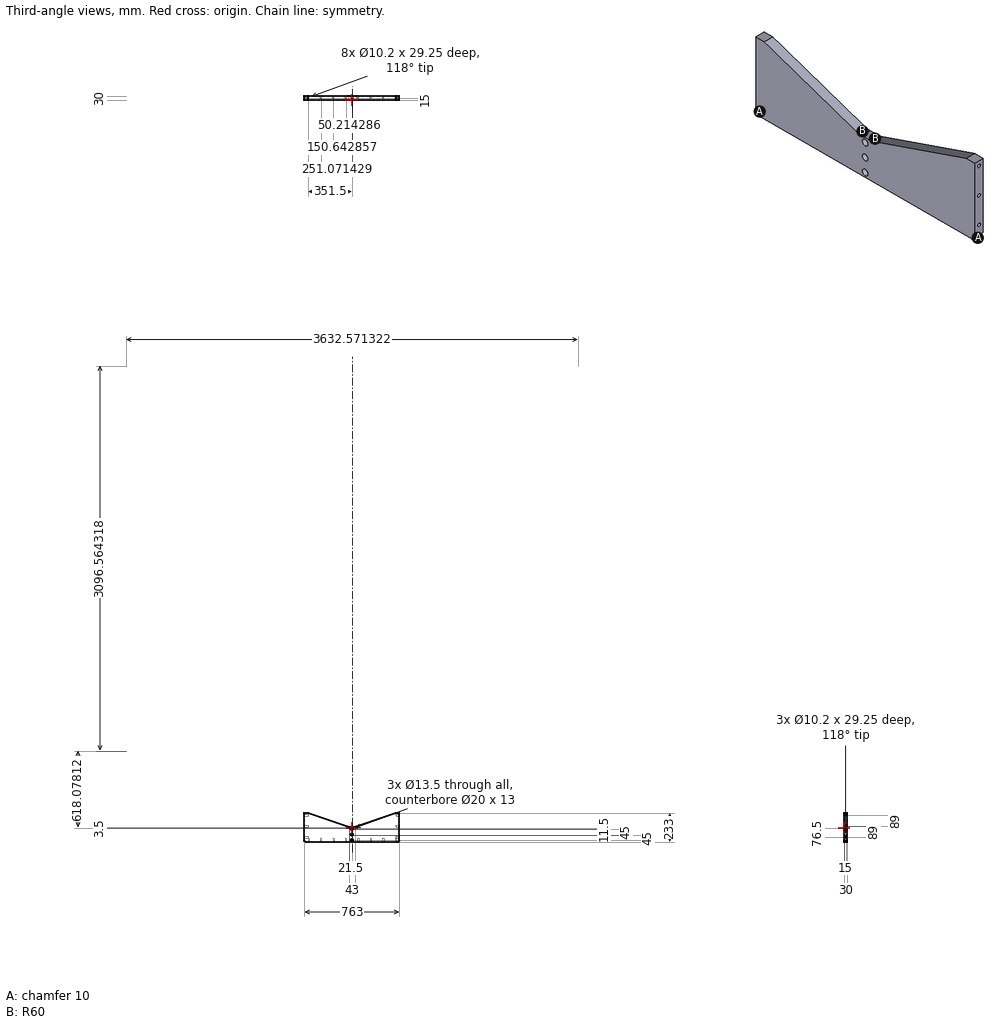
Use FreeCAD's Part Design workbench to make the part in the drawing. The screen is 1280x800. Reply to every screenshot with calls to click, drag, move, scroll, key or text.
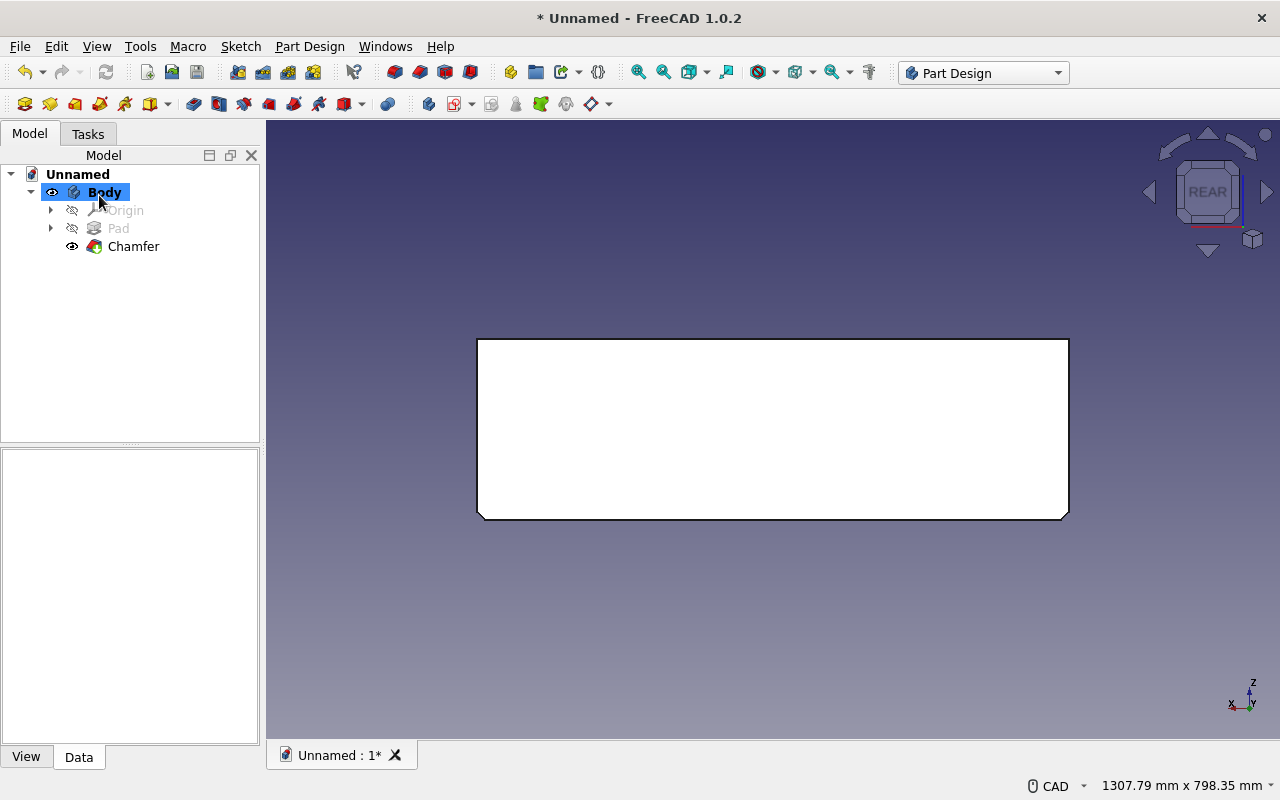
click(604, 428)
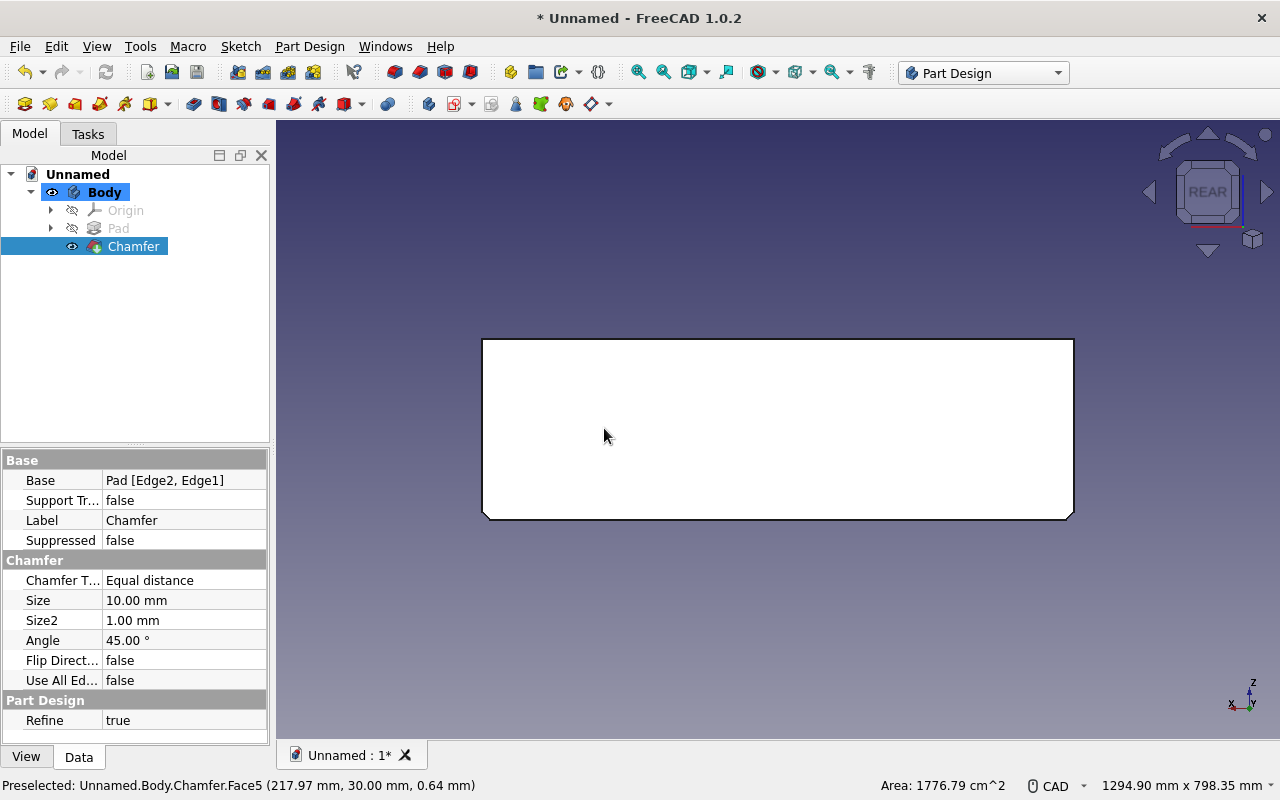
click(454, 104)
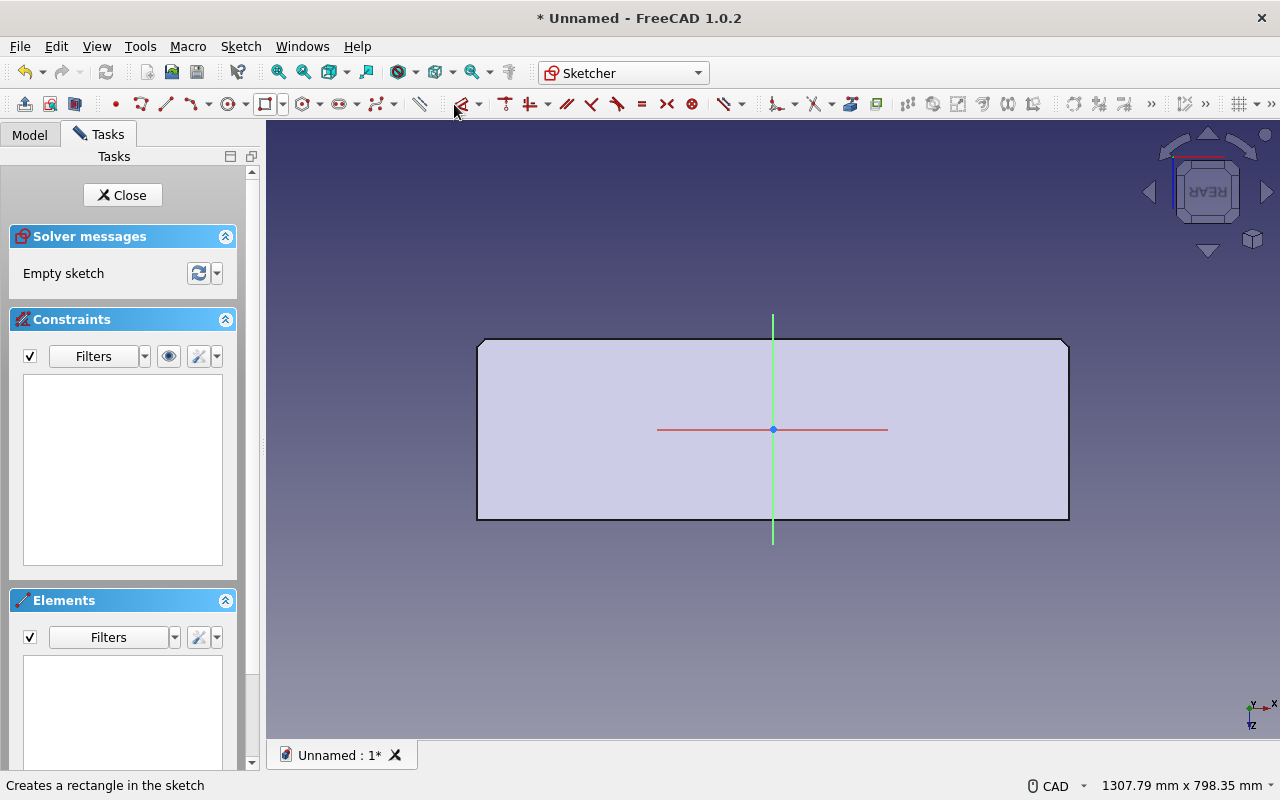
scroll(694, 204, down, 10)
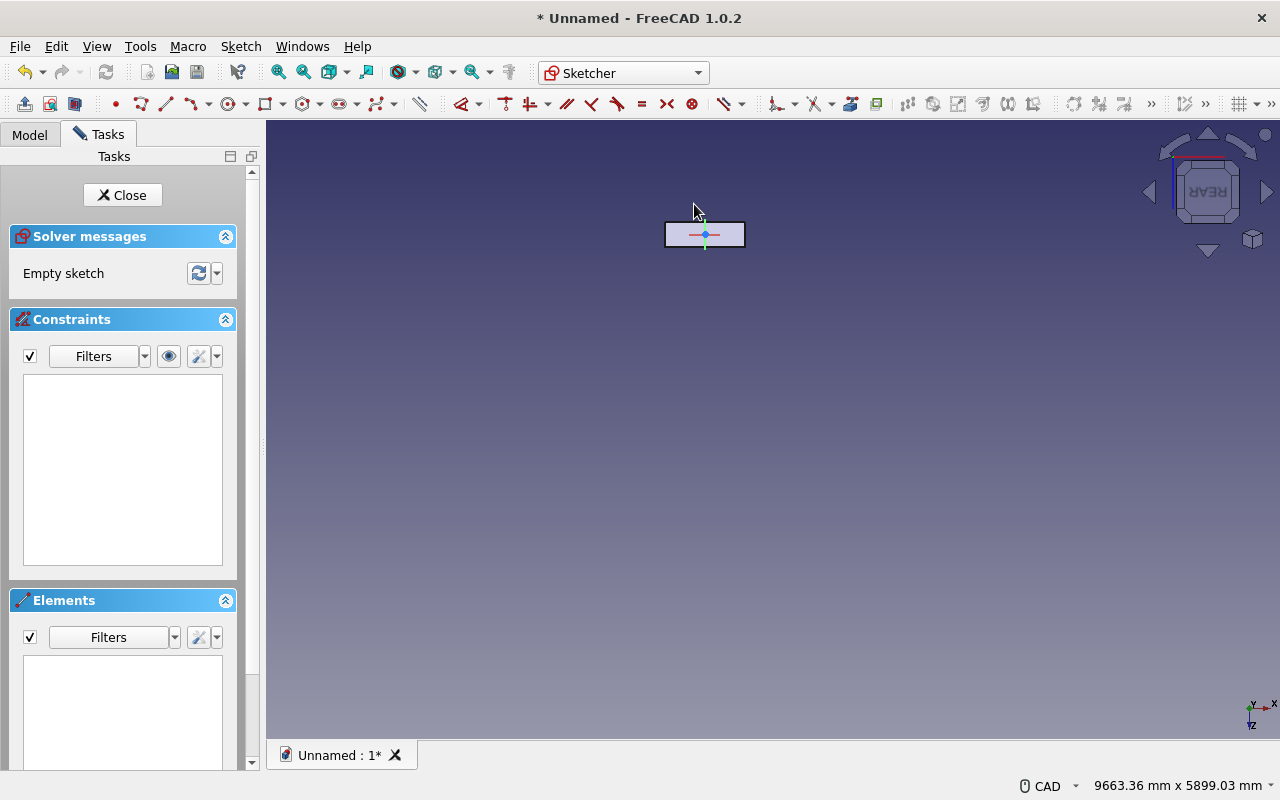
key(g)
key(m)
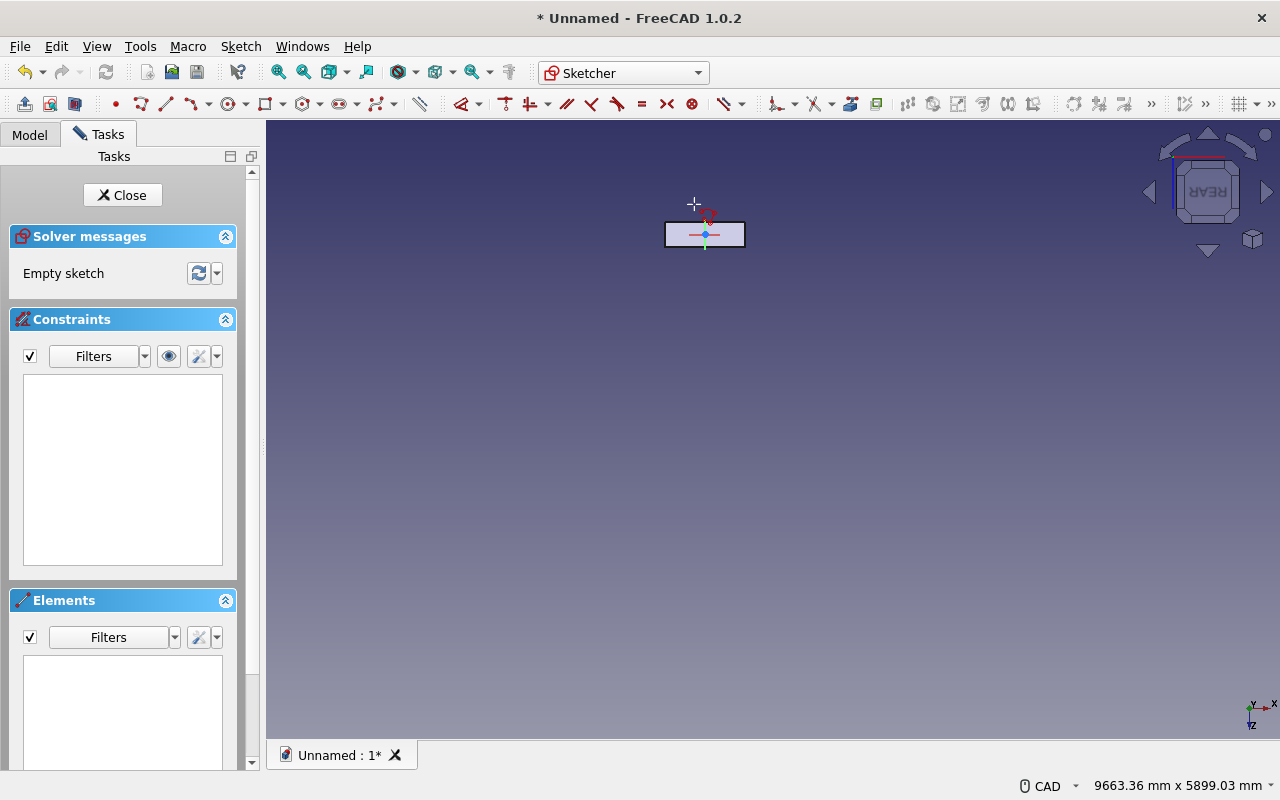
scroll(703, 235, up, 19)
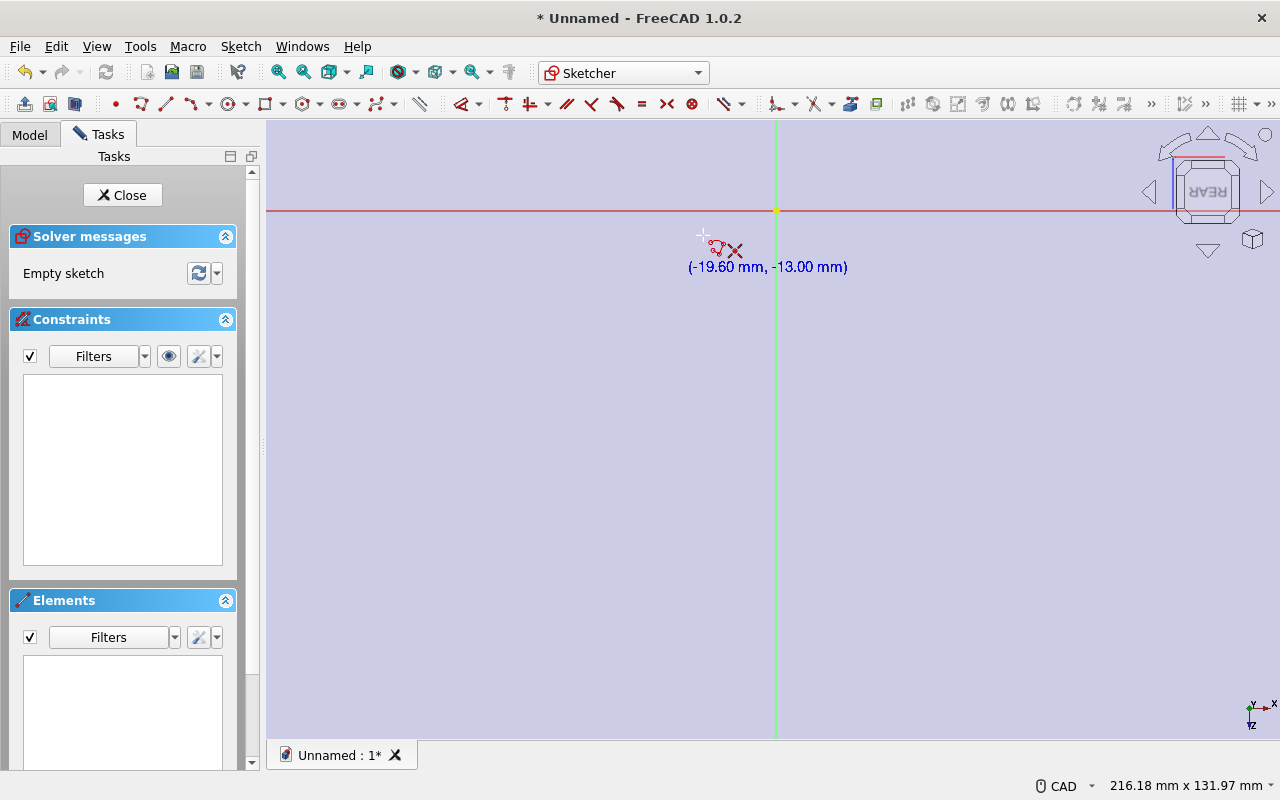
click(675, 227)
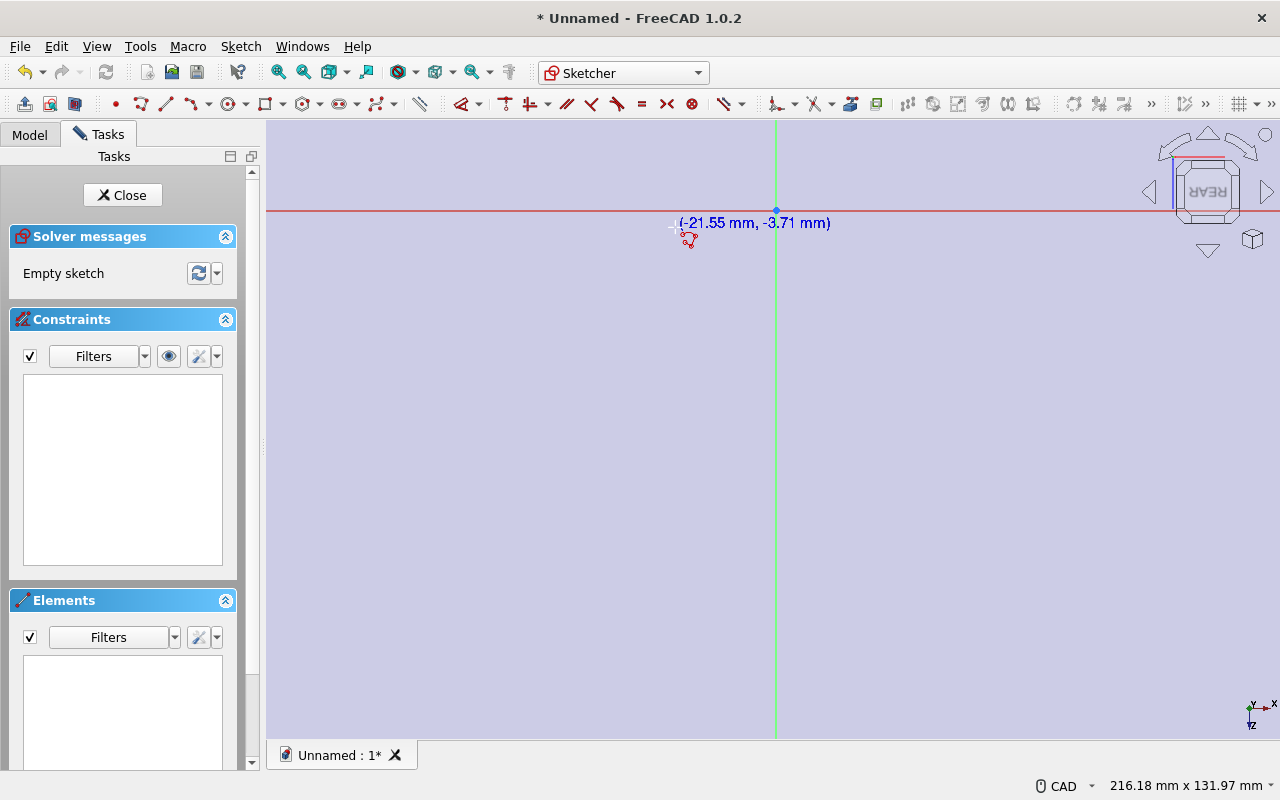
scroll(702, 191, down, 18)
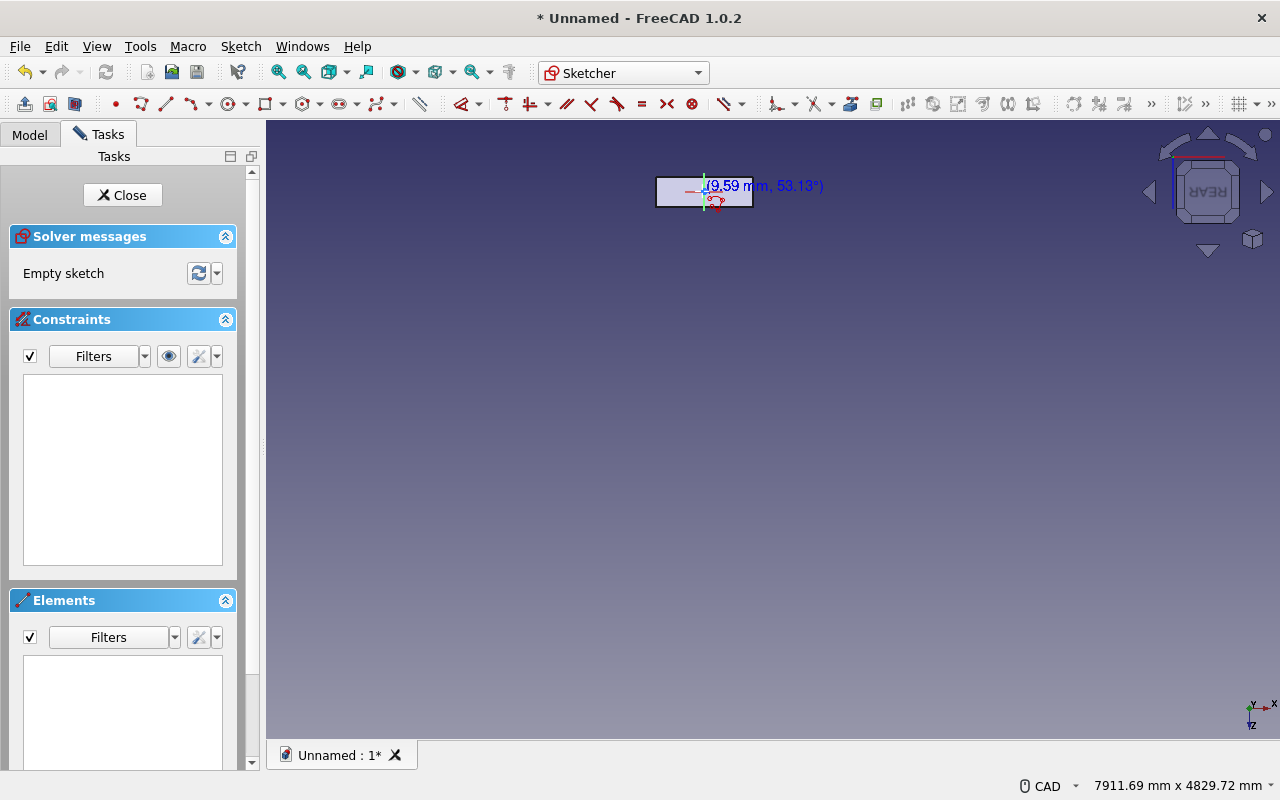
click(472, 271)
click(472, 668)
click(937, 668)
click(937, 271)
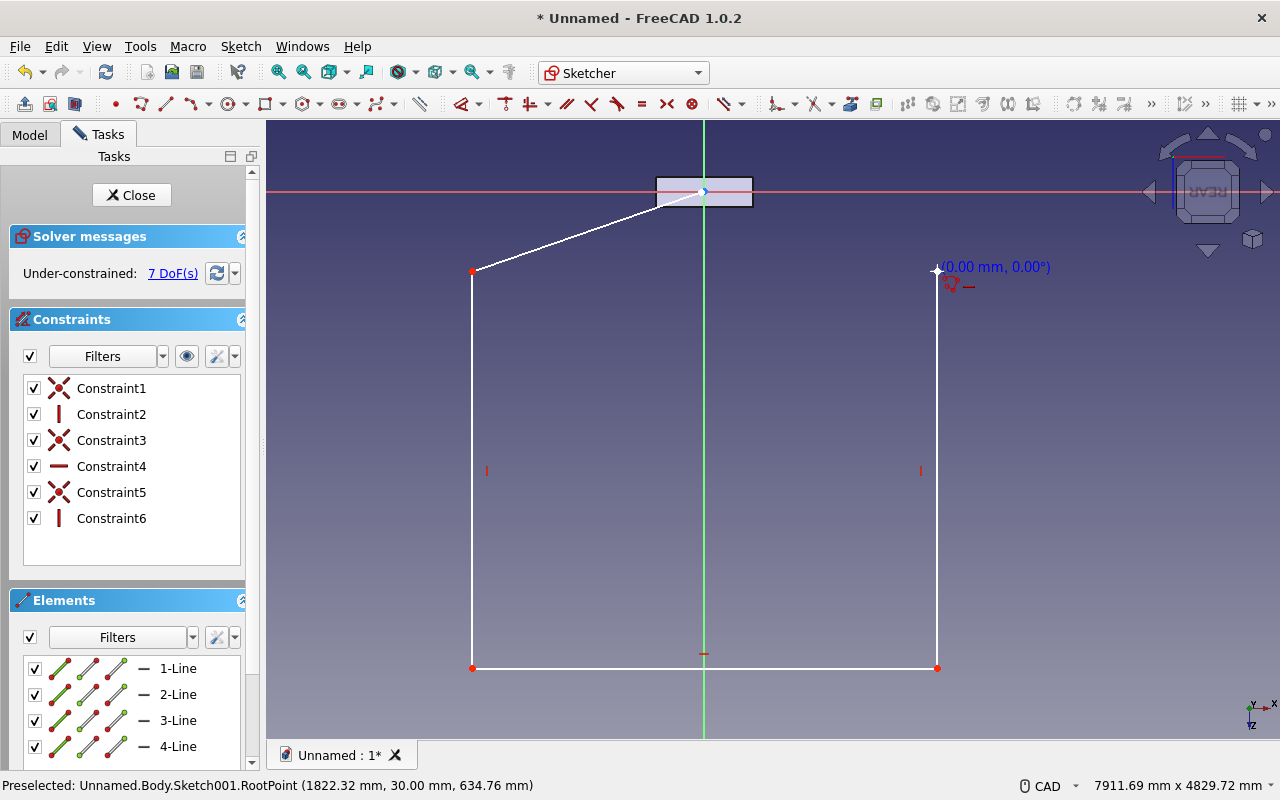
scroll(707, 192, up, 18)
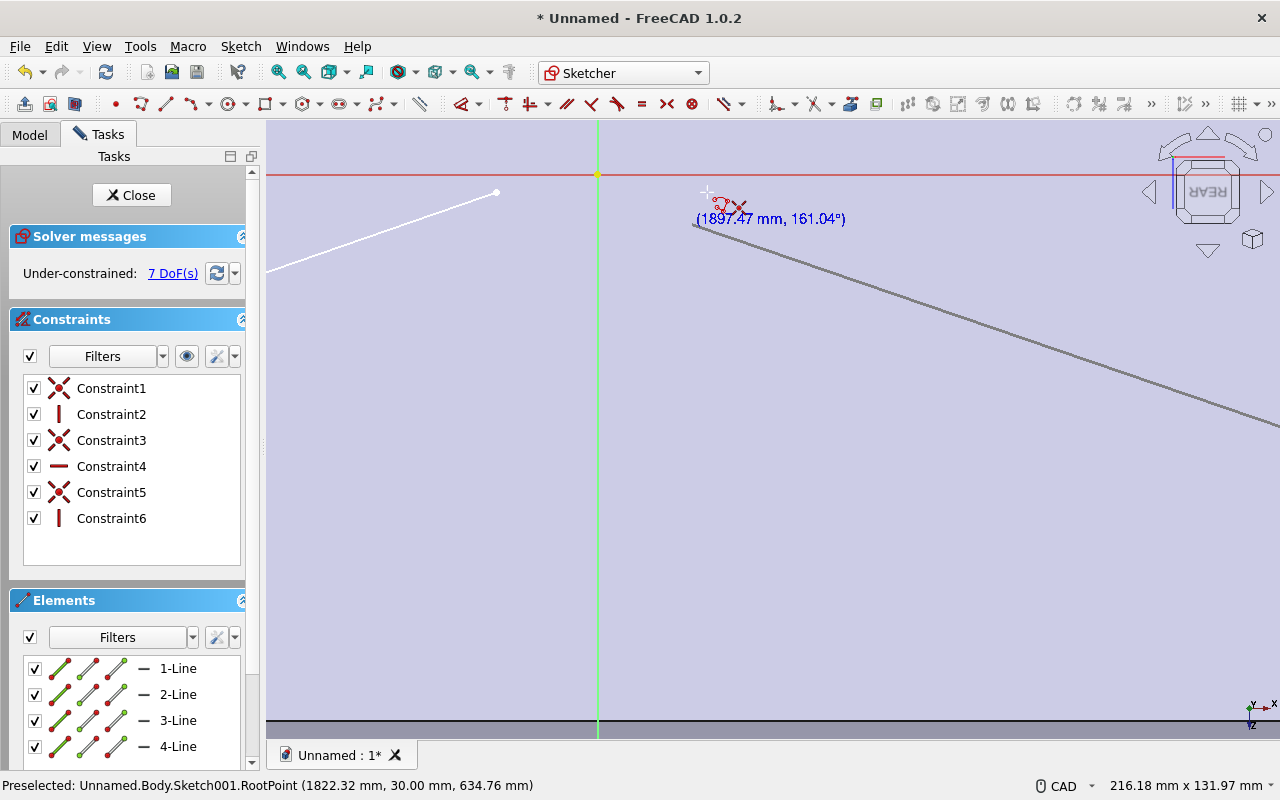
click(699, 191)
click(497, 192)
key(Escape)
key(Escape)